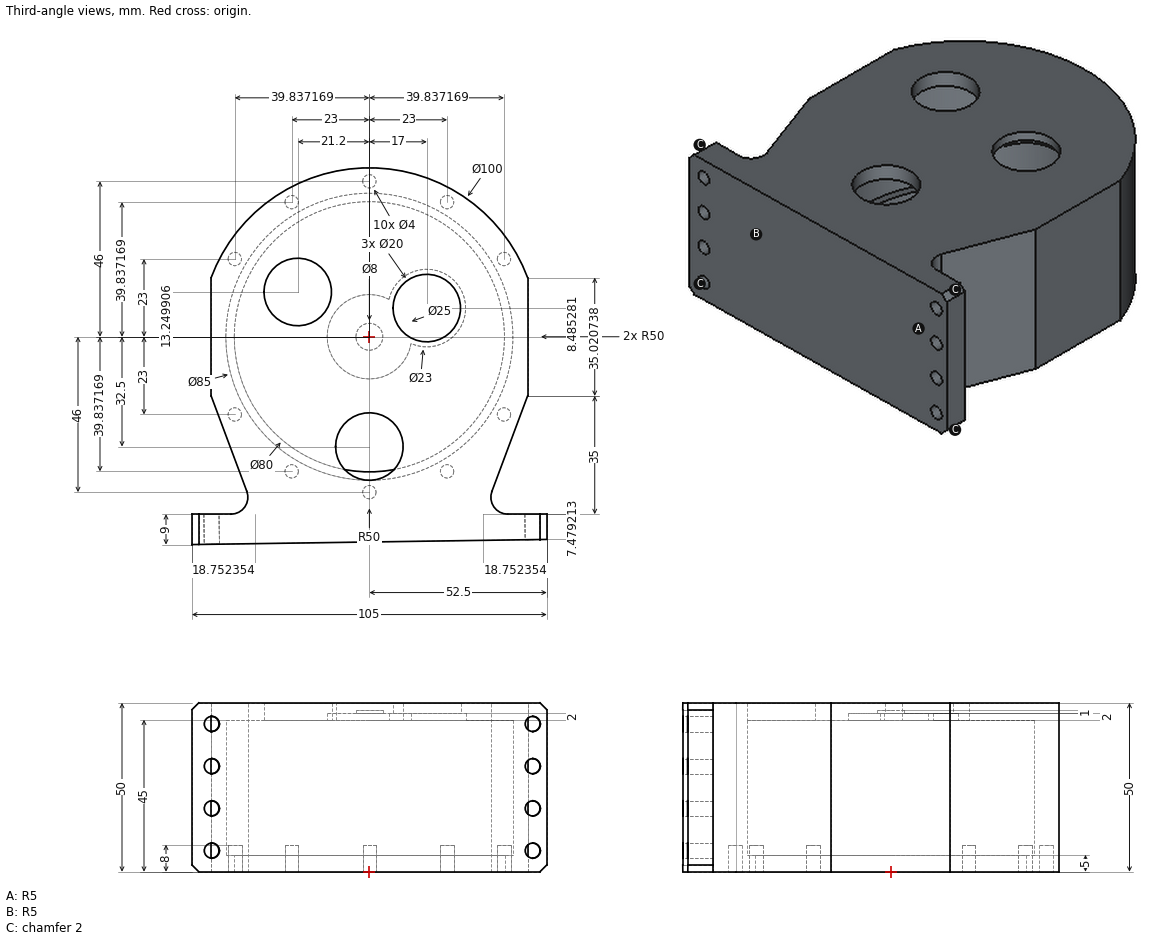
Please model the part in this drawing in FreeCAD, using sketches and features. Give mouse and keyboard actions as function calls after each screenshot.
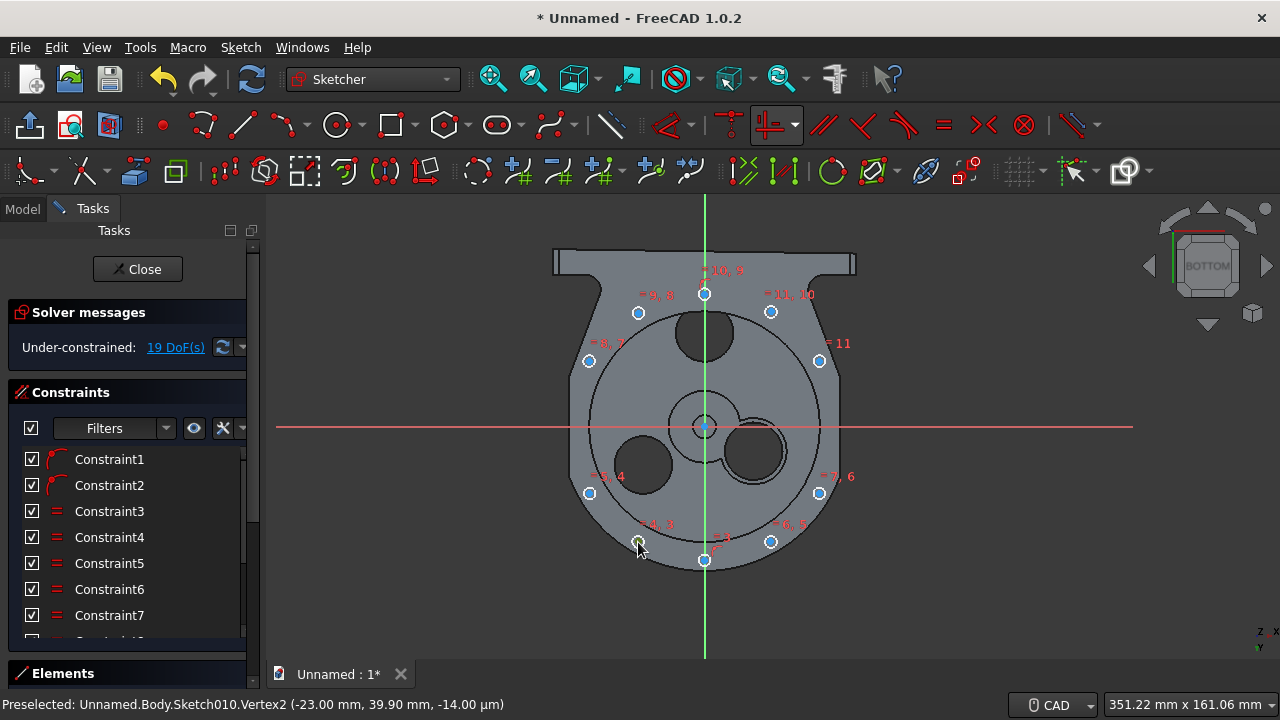
click(771, 542)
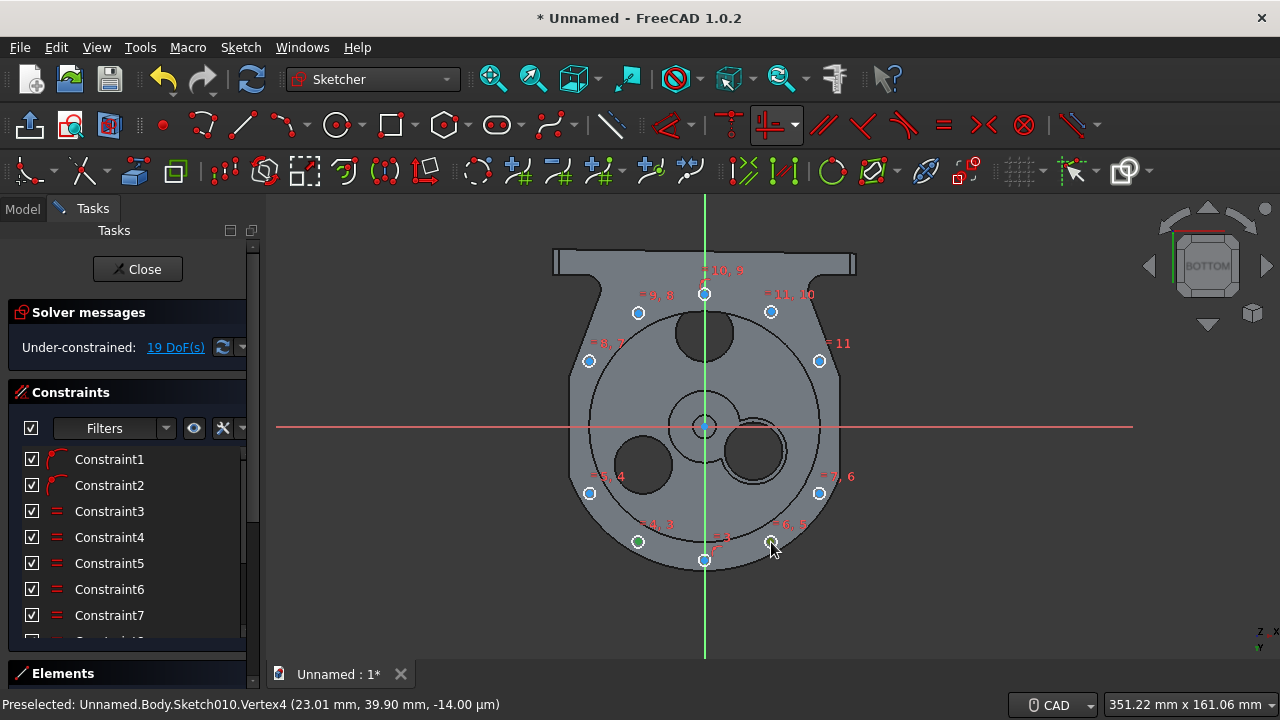
key(h)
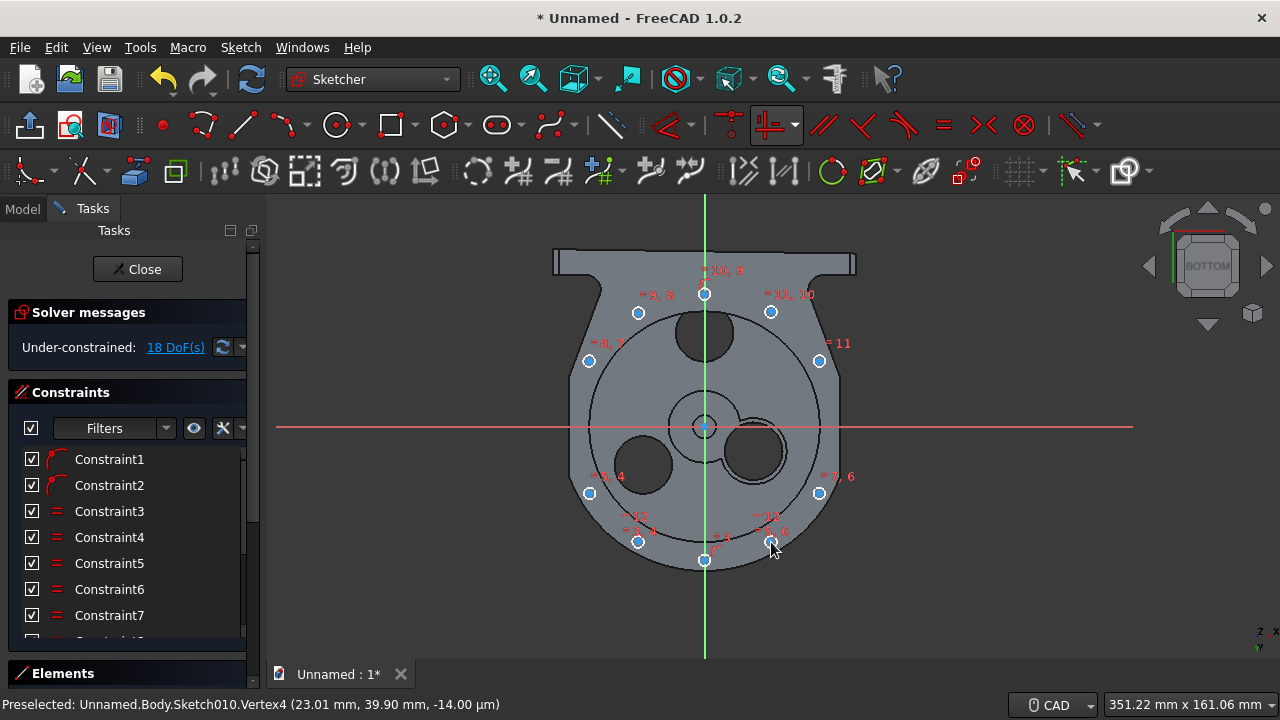
click(590, 493)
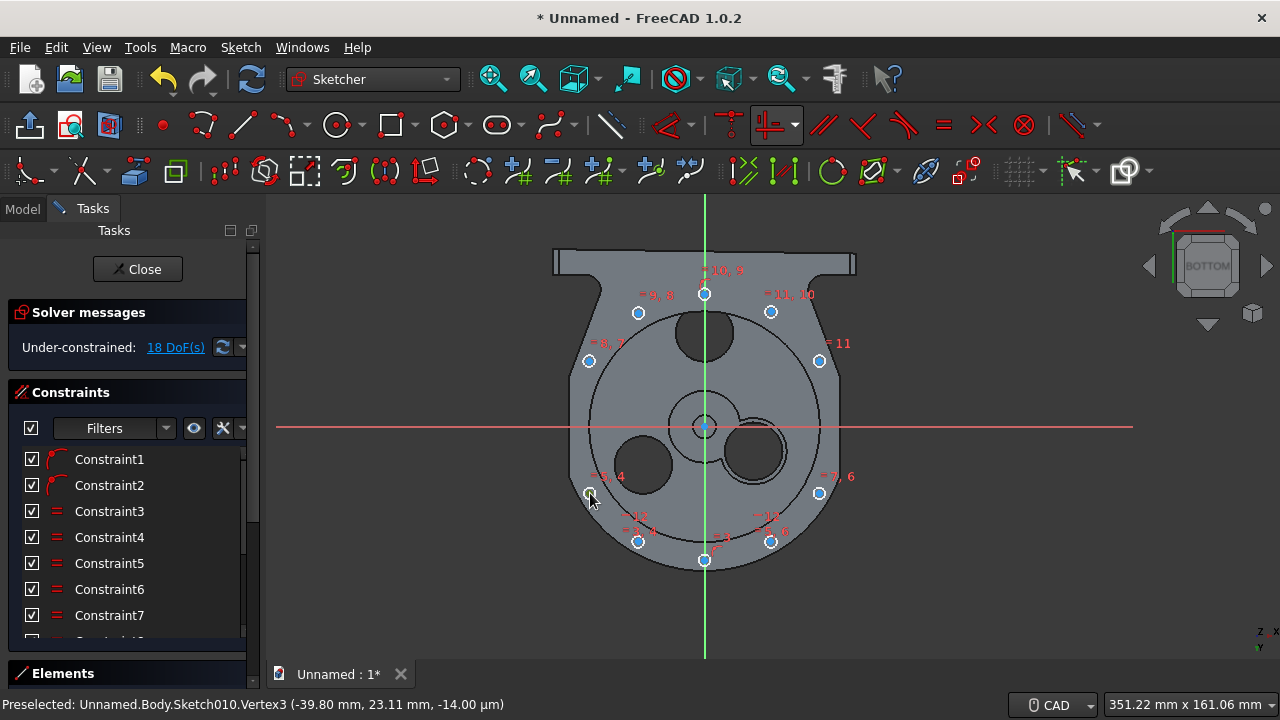
click(819, 493)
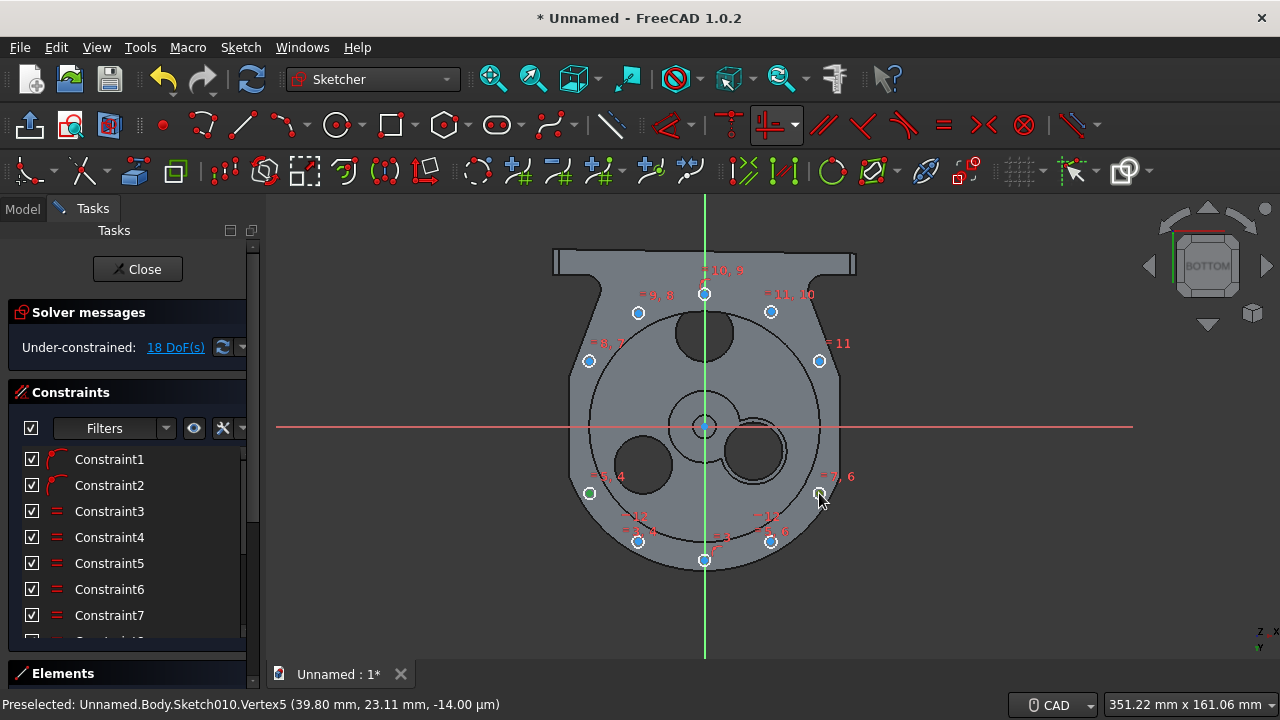
key(h)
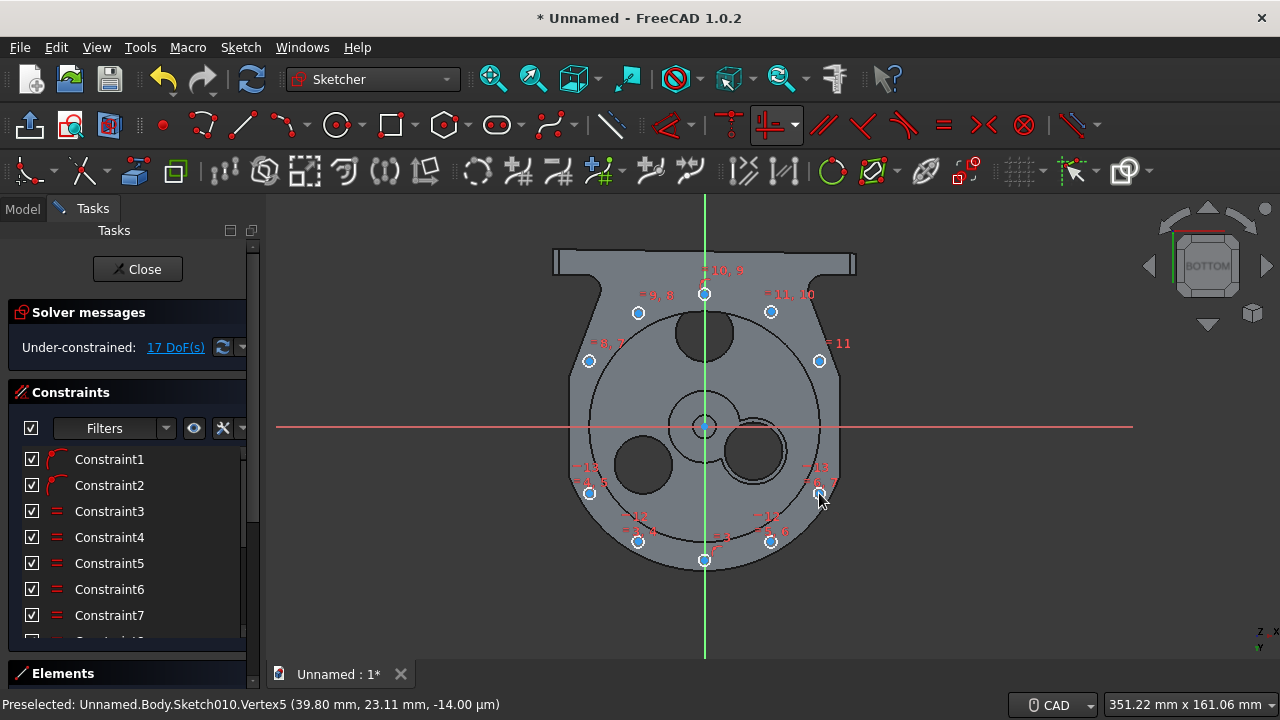
click(590, 493)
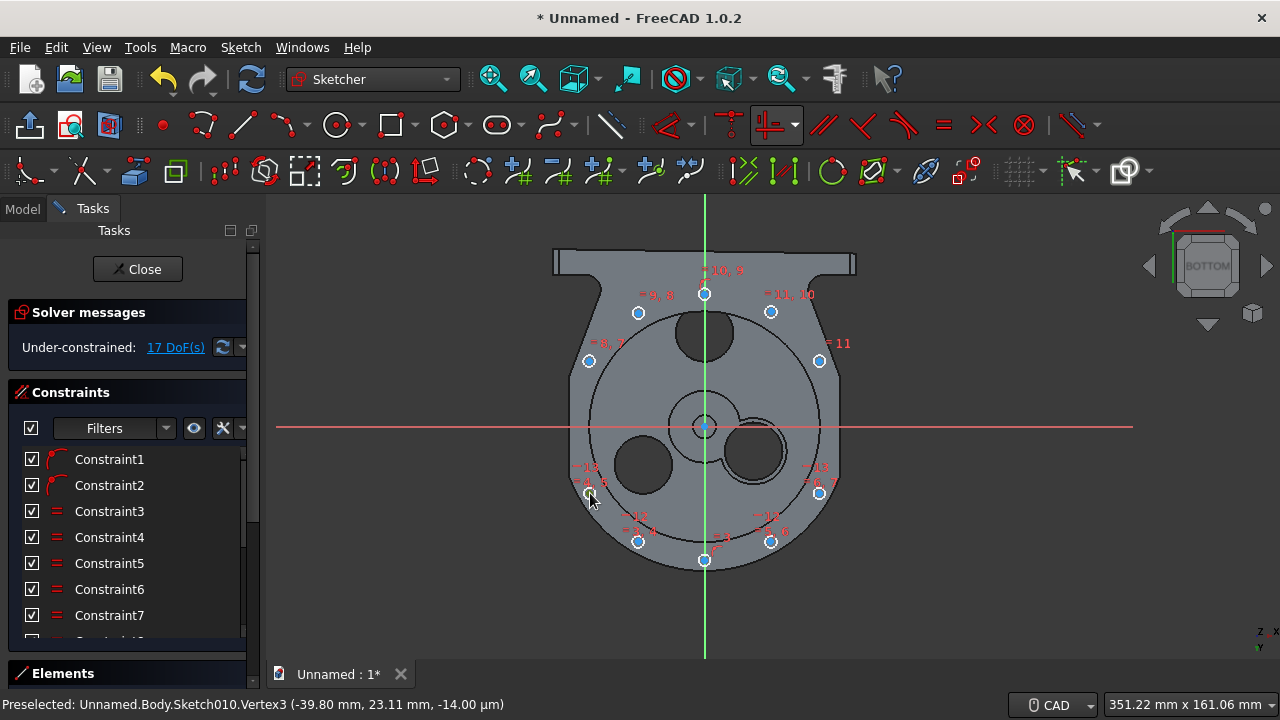
click(589, 361)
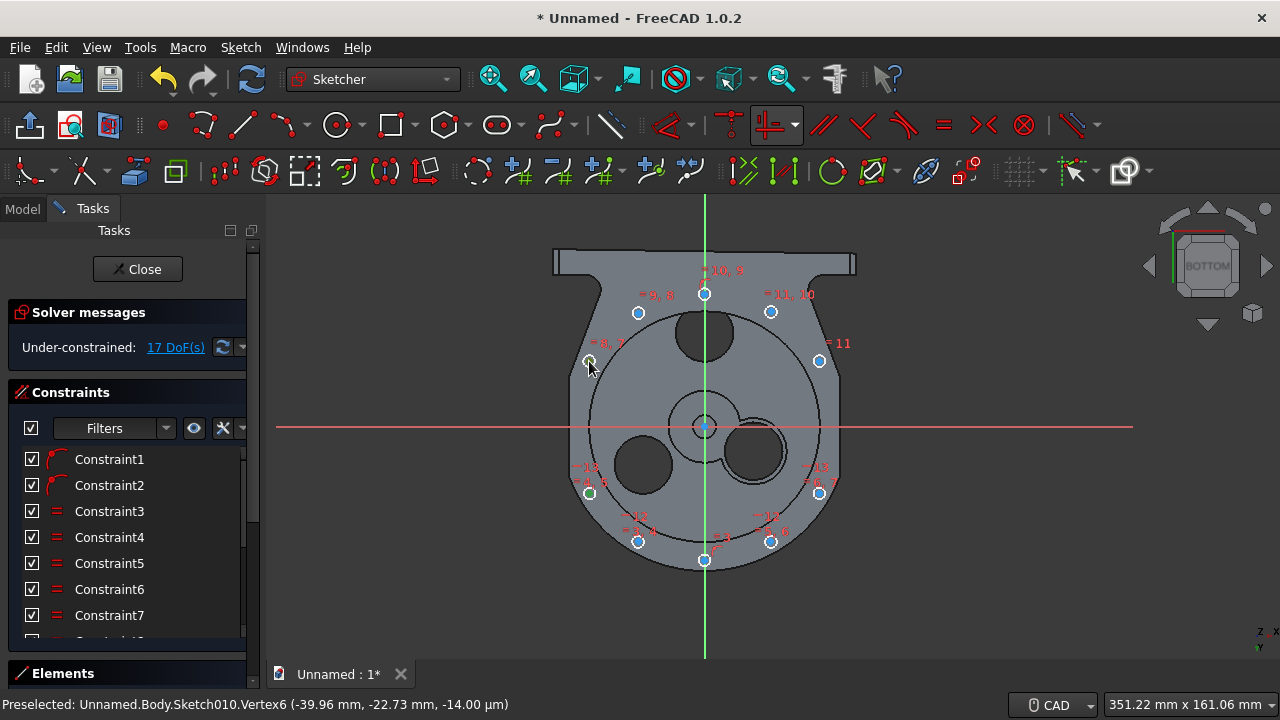
click(798, 126)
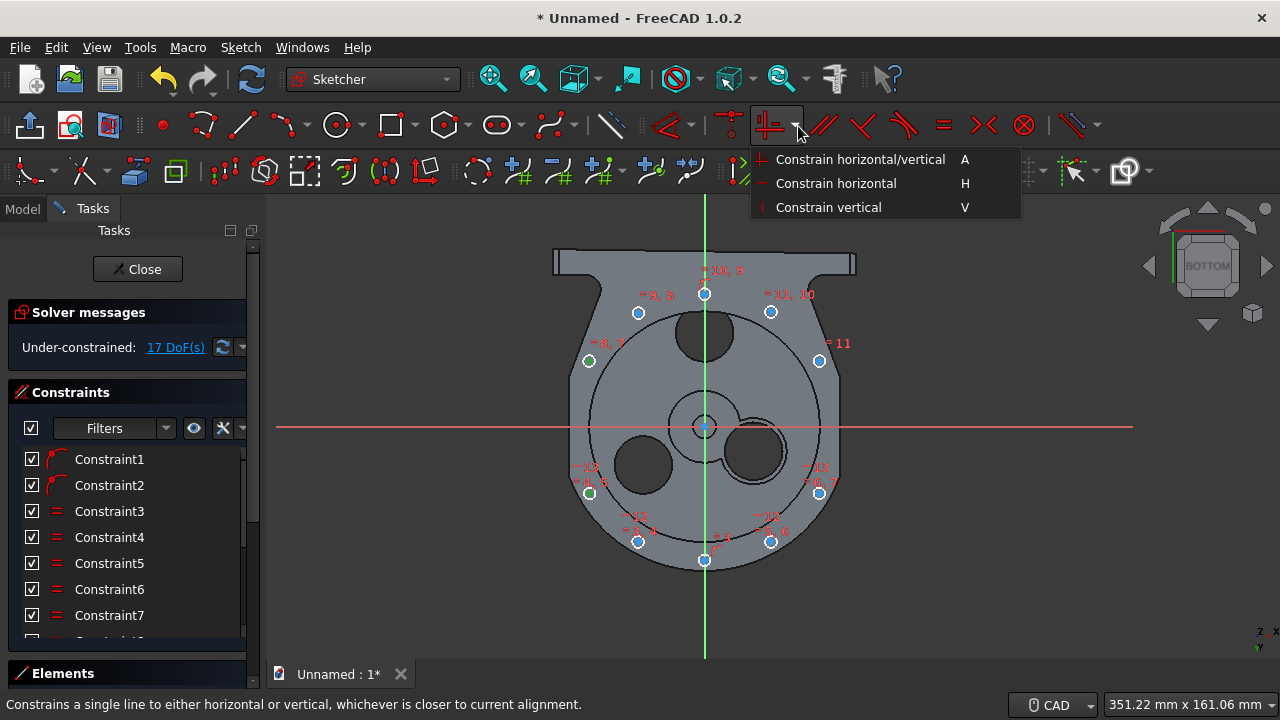
click(886, 207)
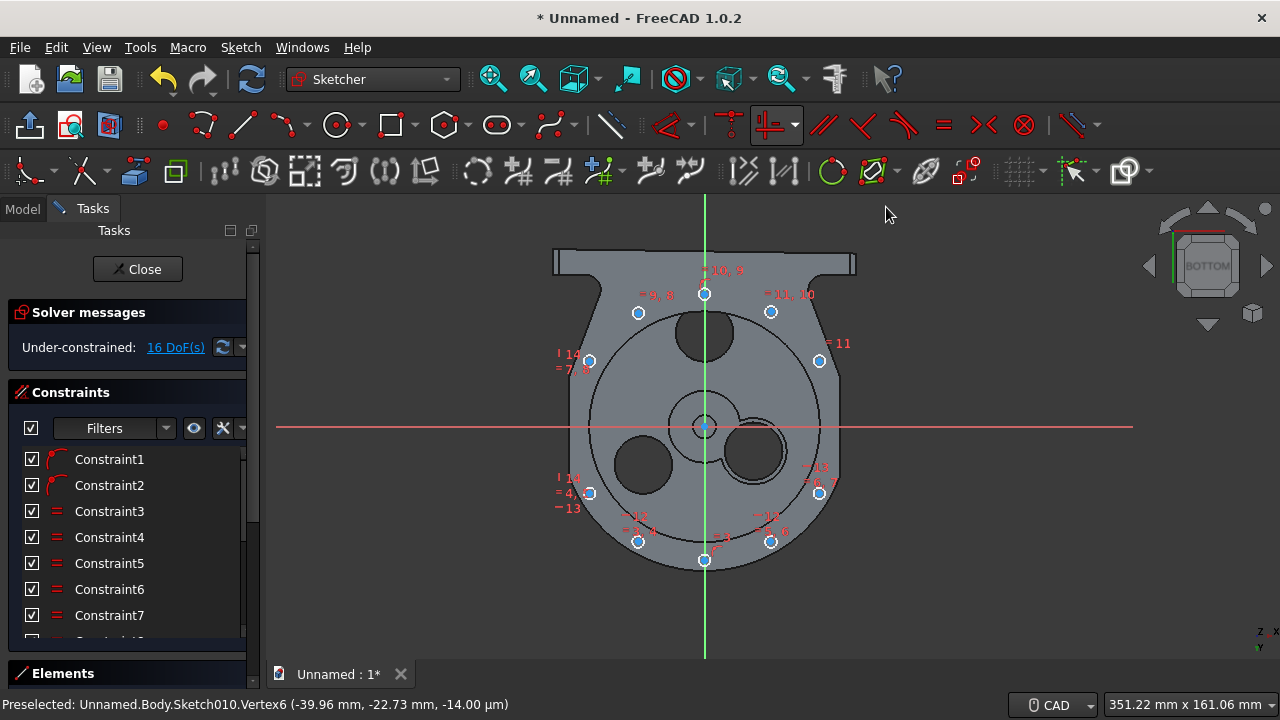
click(638, 542)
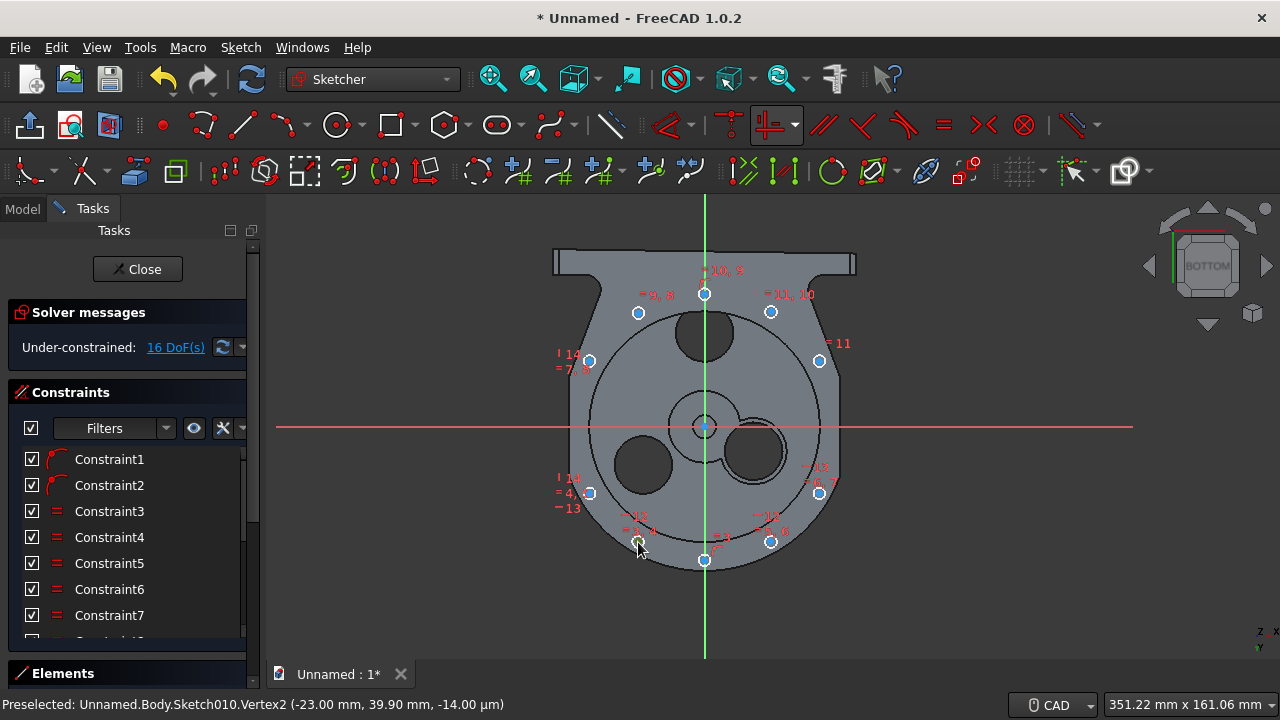
click(638, 313)